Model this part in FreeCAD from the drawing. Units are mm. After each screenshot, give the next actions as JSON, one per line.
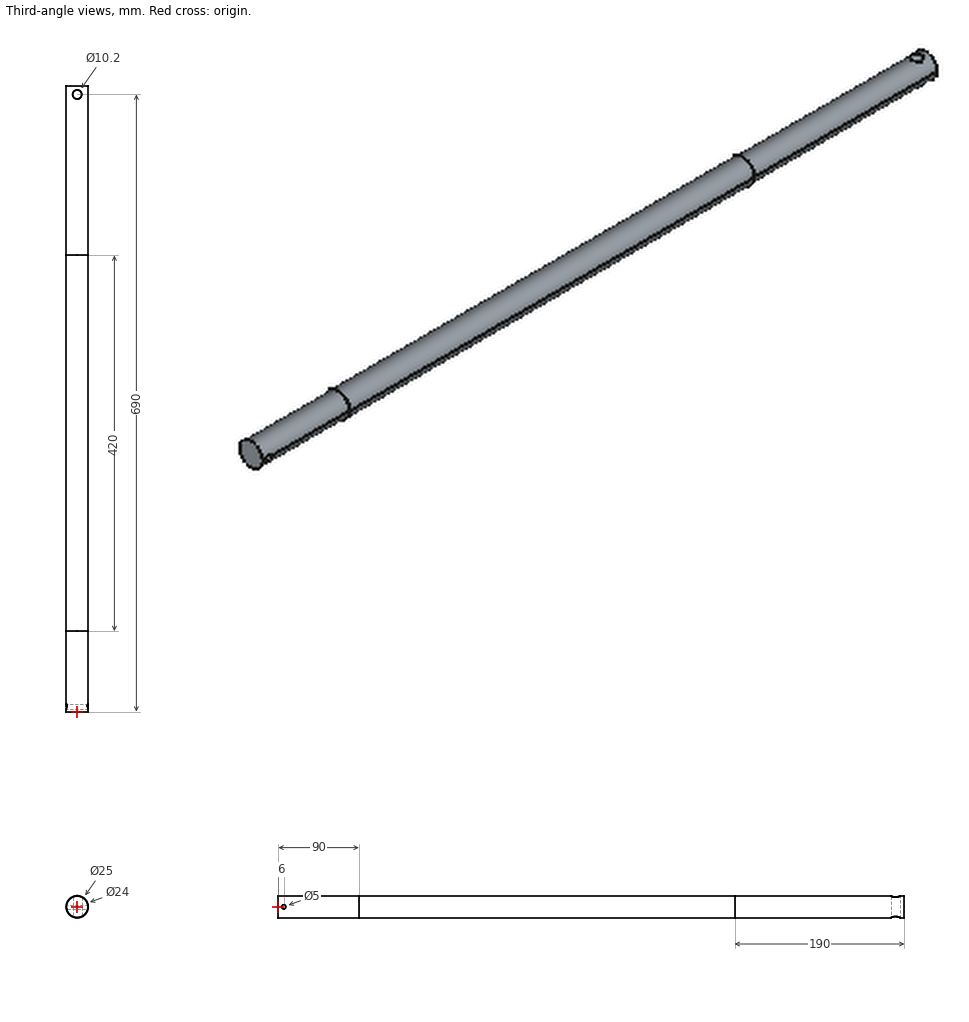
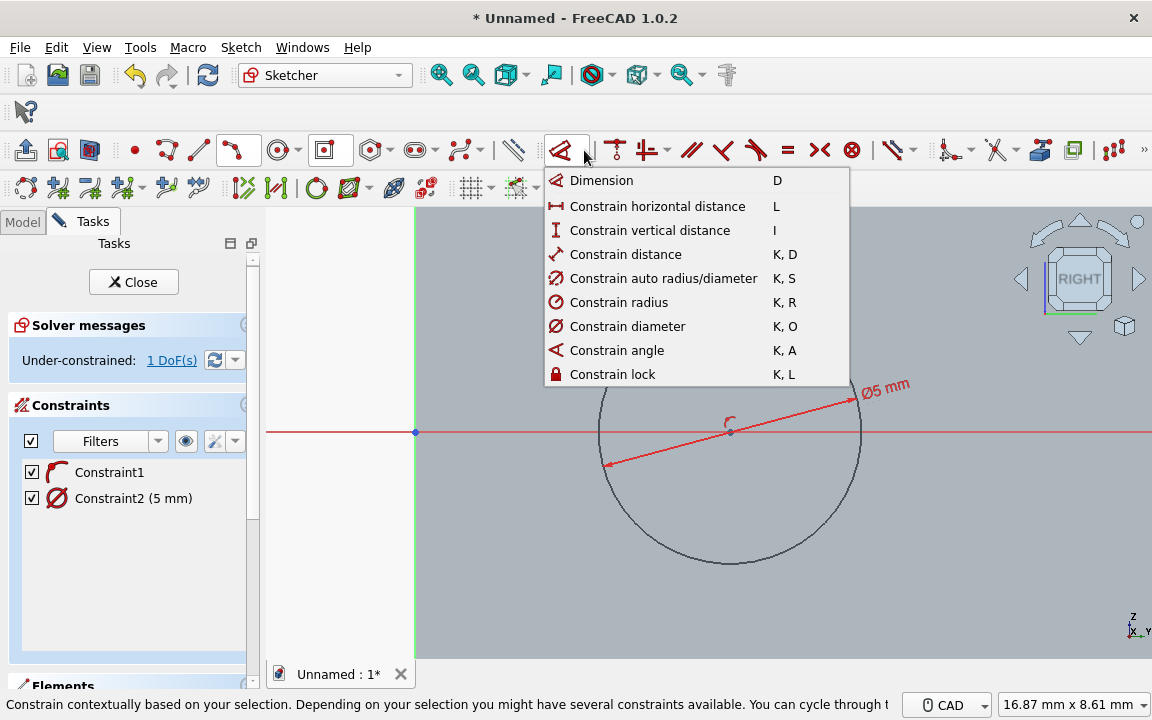
{"action": "left_click", "coordinate": [697, 206]}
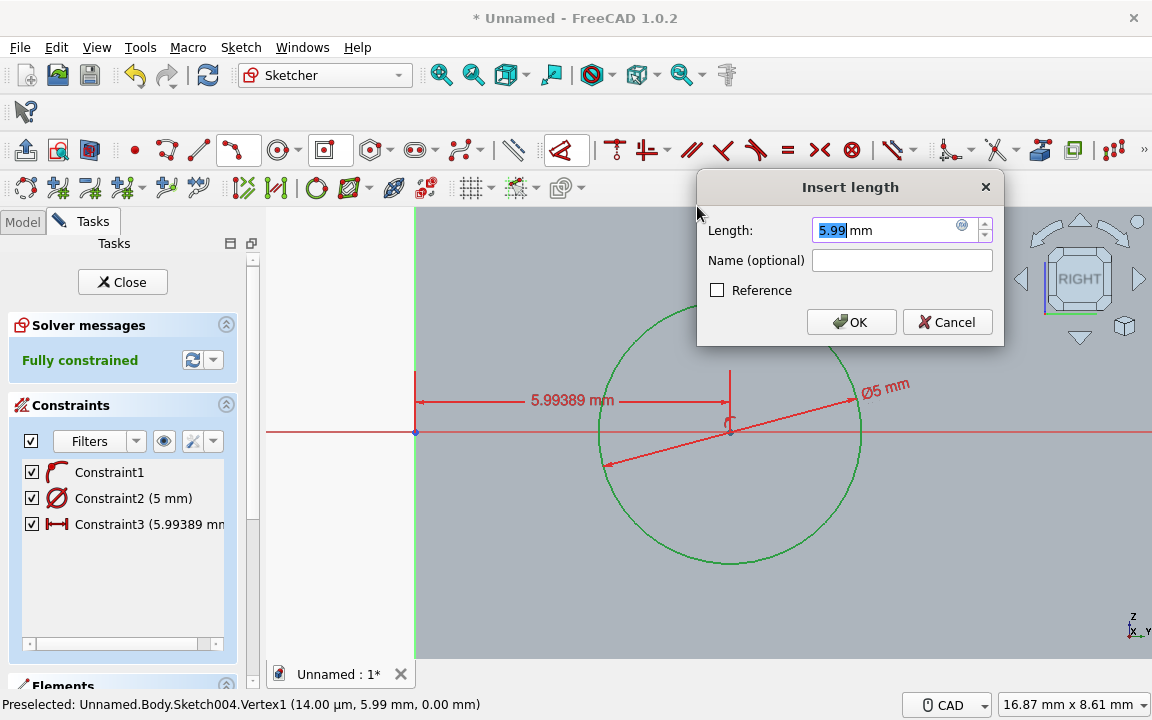
{"action": "type", "text": "6"}
{"action": "key", "text": "Return"}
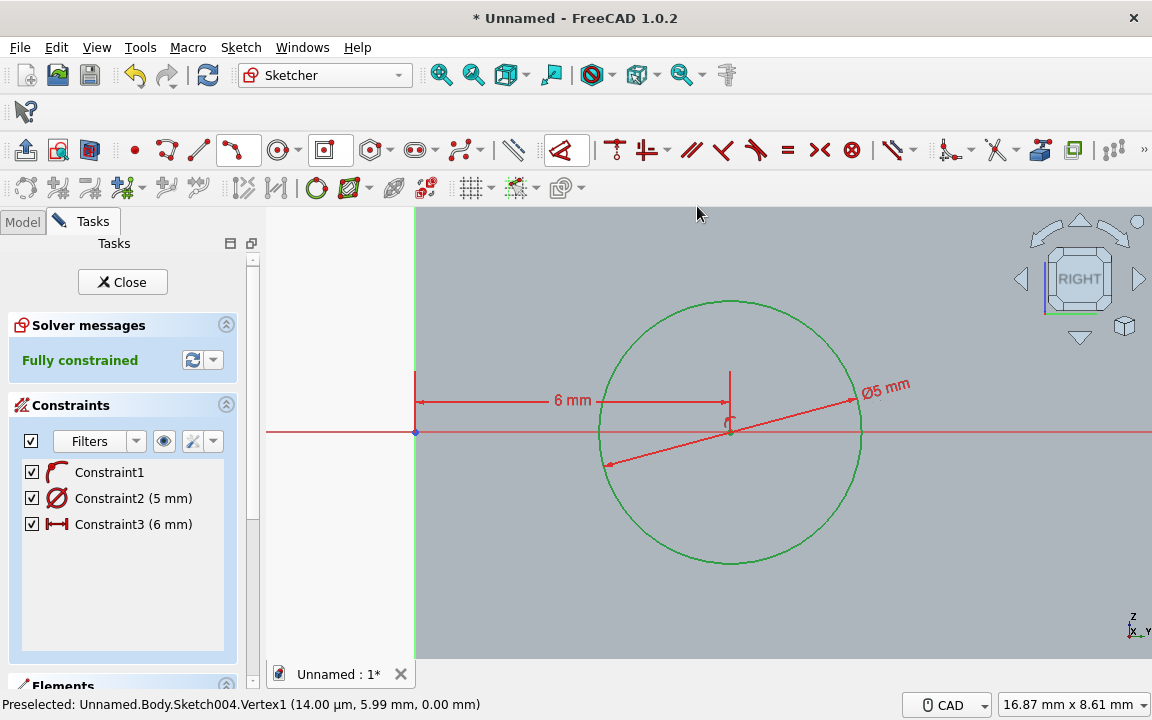
{"action": "left_click", "coordinate": [123, 282]}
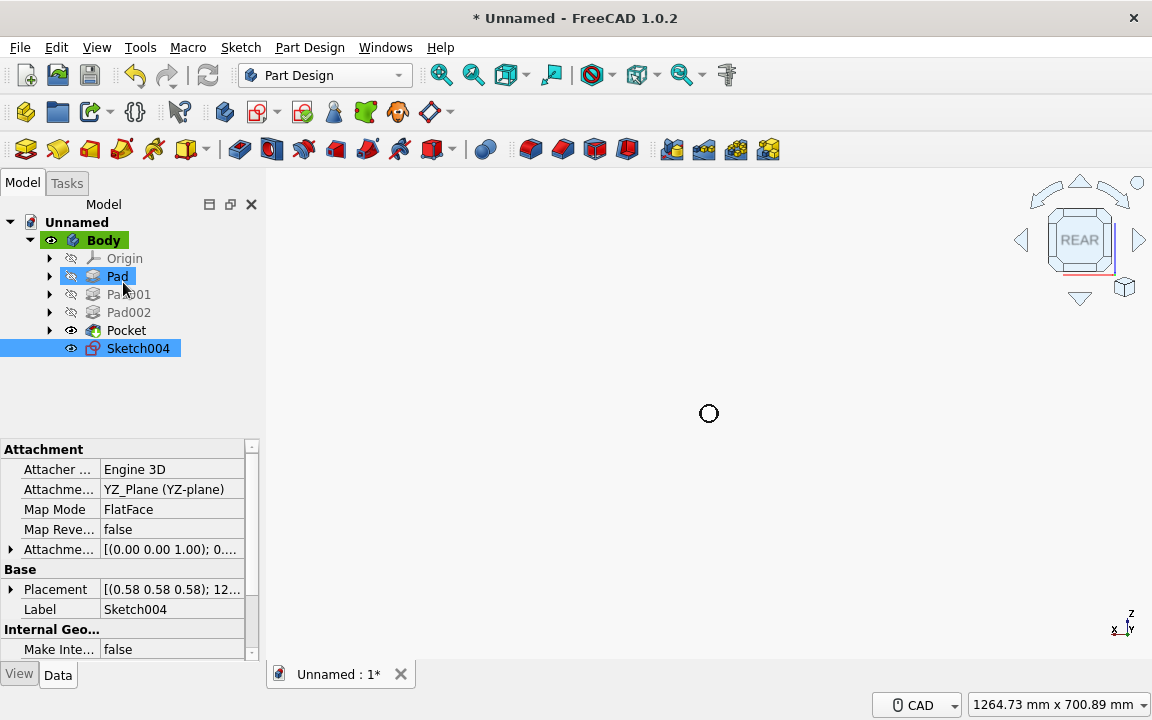
{"action": "left_click", "coordinate": [240, 150]}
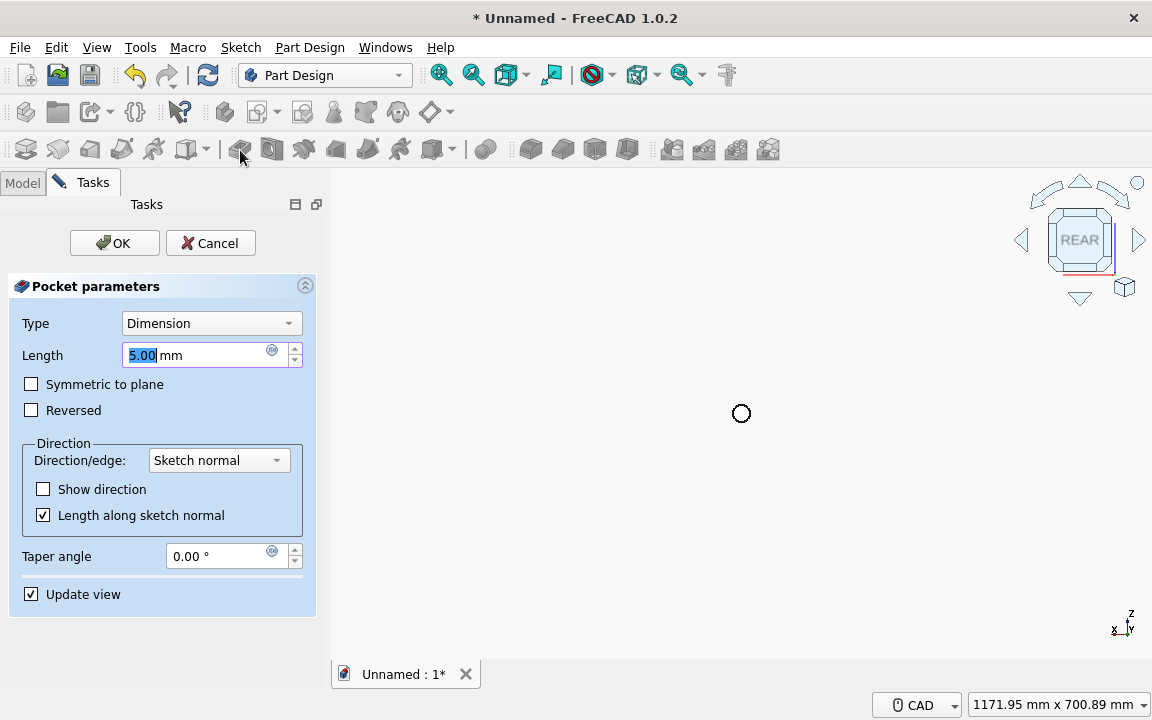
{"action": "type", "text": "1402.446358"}
{"action": "key", "text": "Tab"}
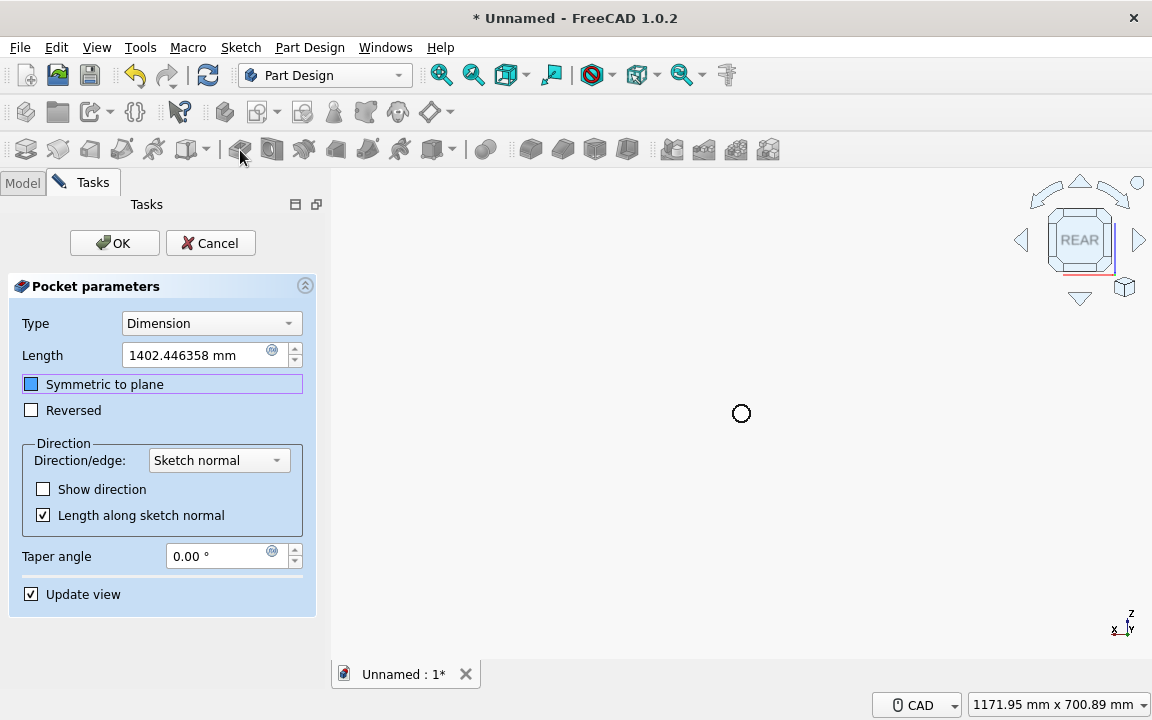
{"action": "left_click", "coordinate": [30, 384]}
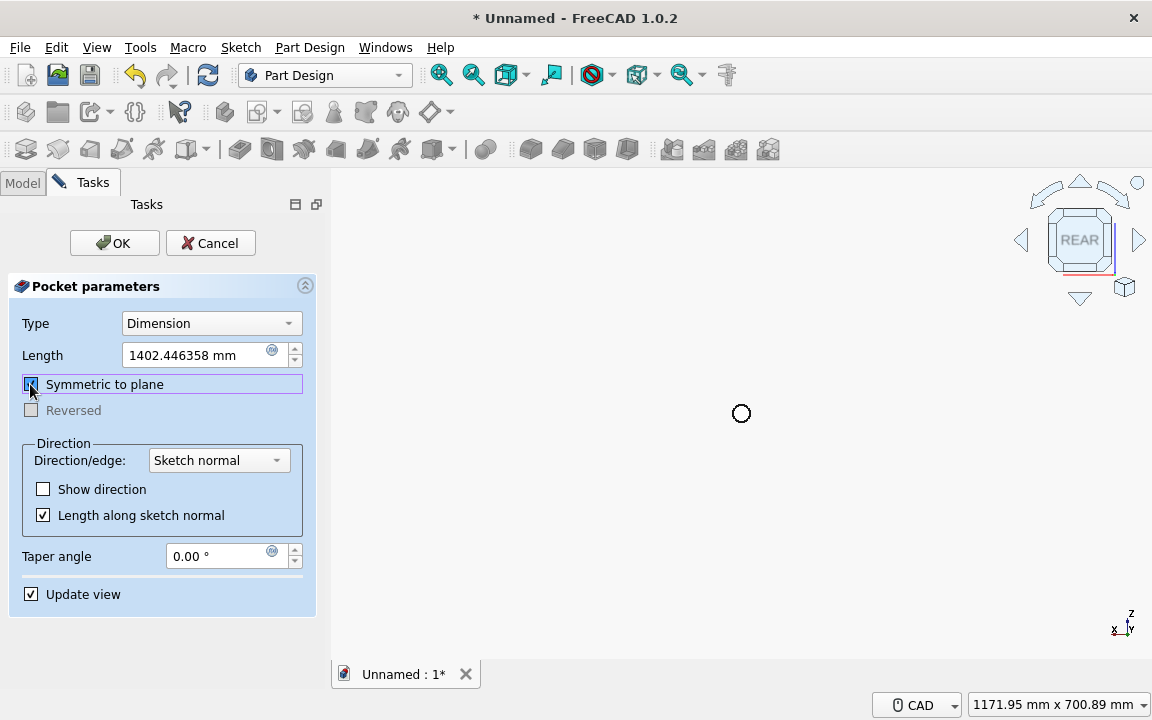
{"action": "left_click", "coordinate": [115, 243]}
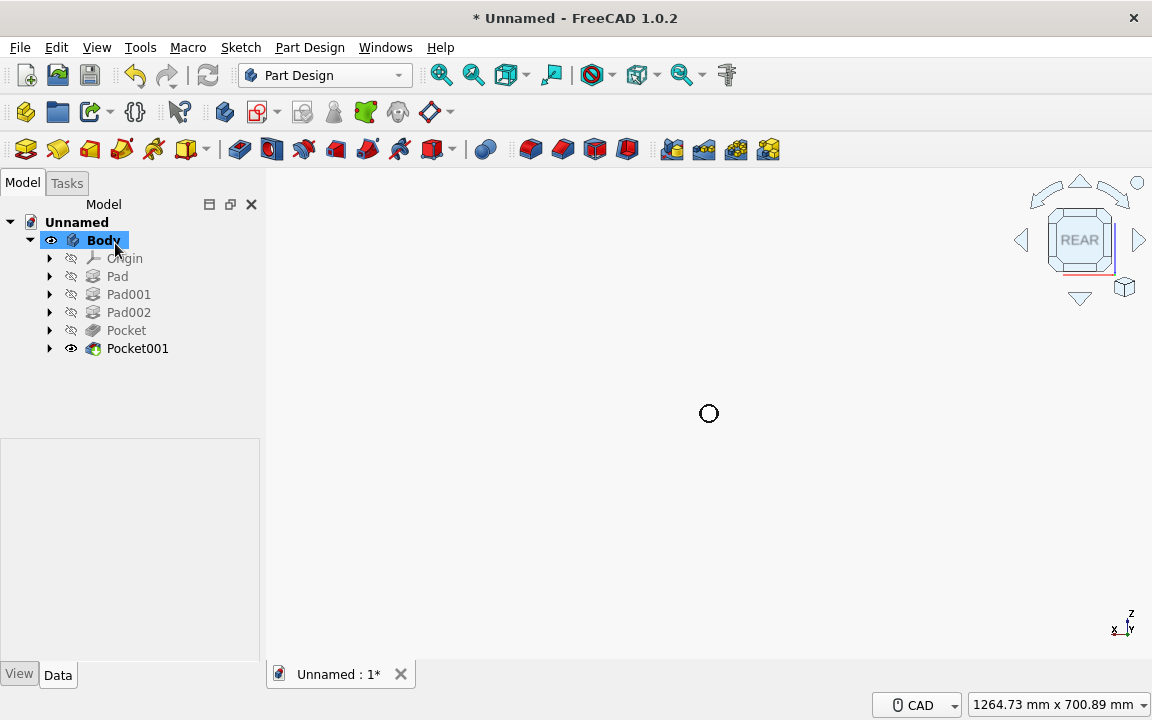
{"action": "key", "text": "0"}